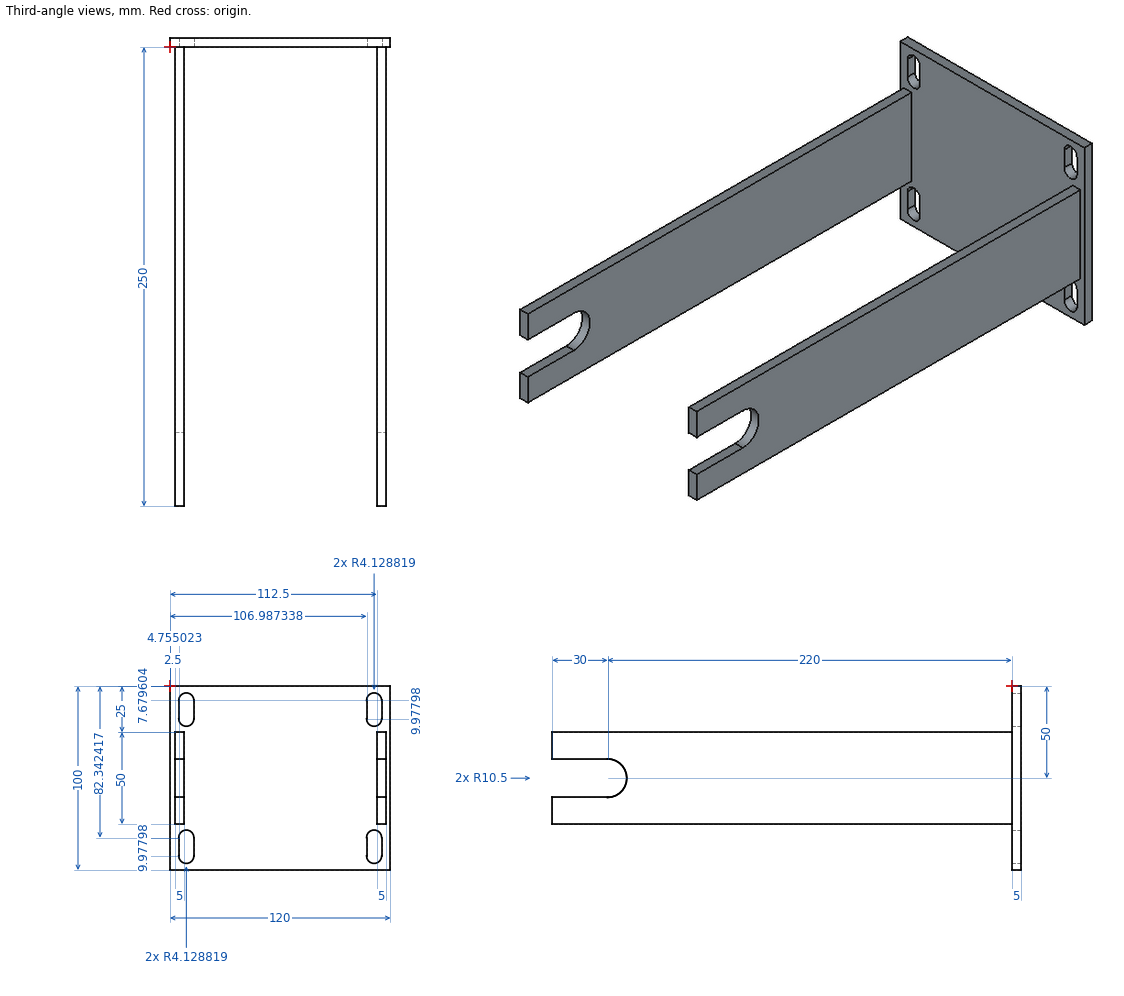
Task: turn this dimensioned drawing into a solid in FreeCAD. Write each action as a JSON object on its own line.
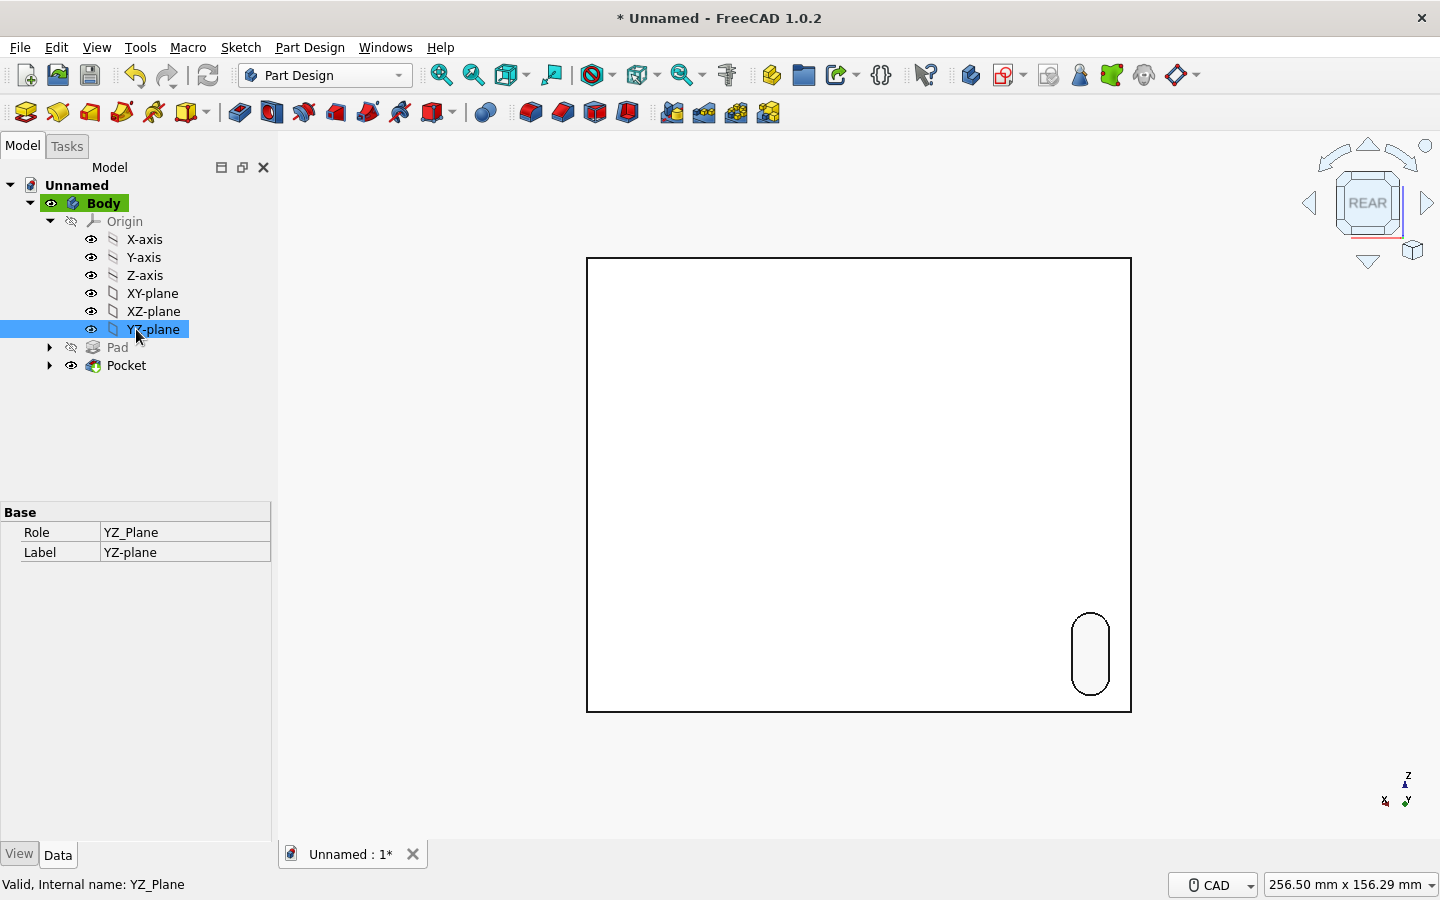
{"action": "left_click", "coordinate": [1176, 76]}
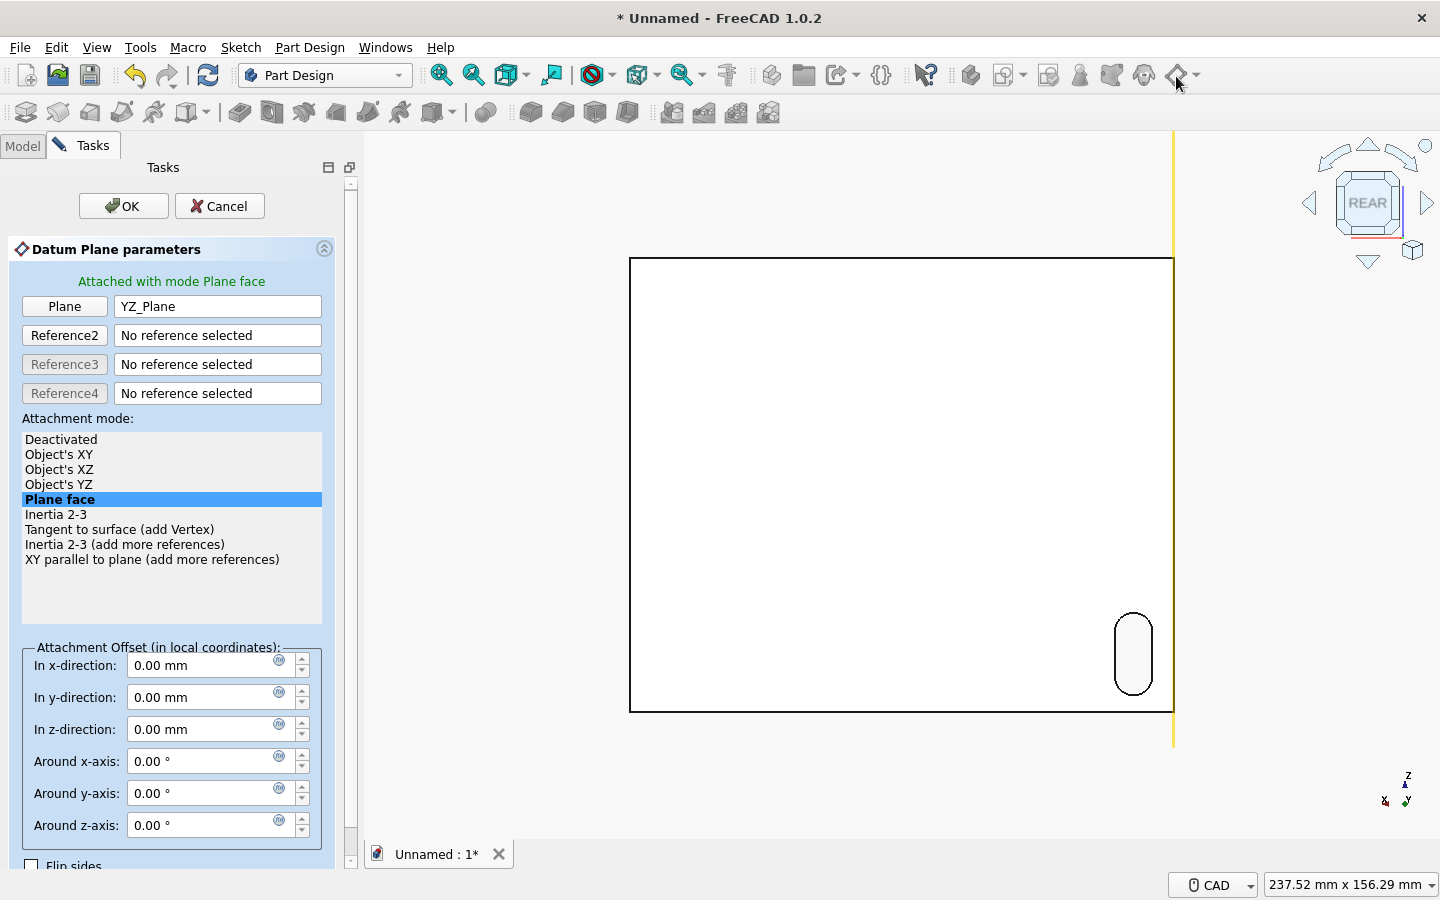
{"action": "triple_click", "coordinate": [210, 729]}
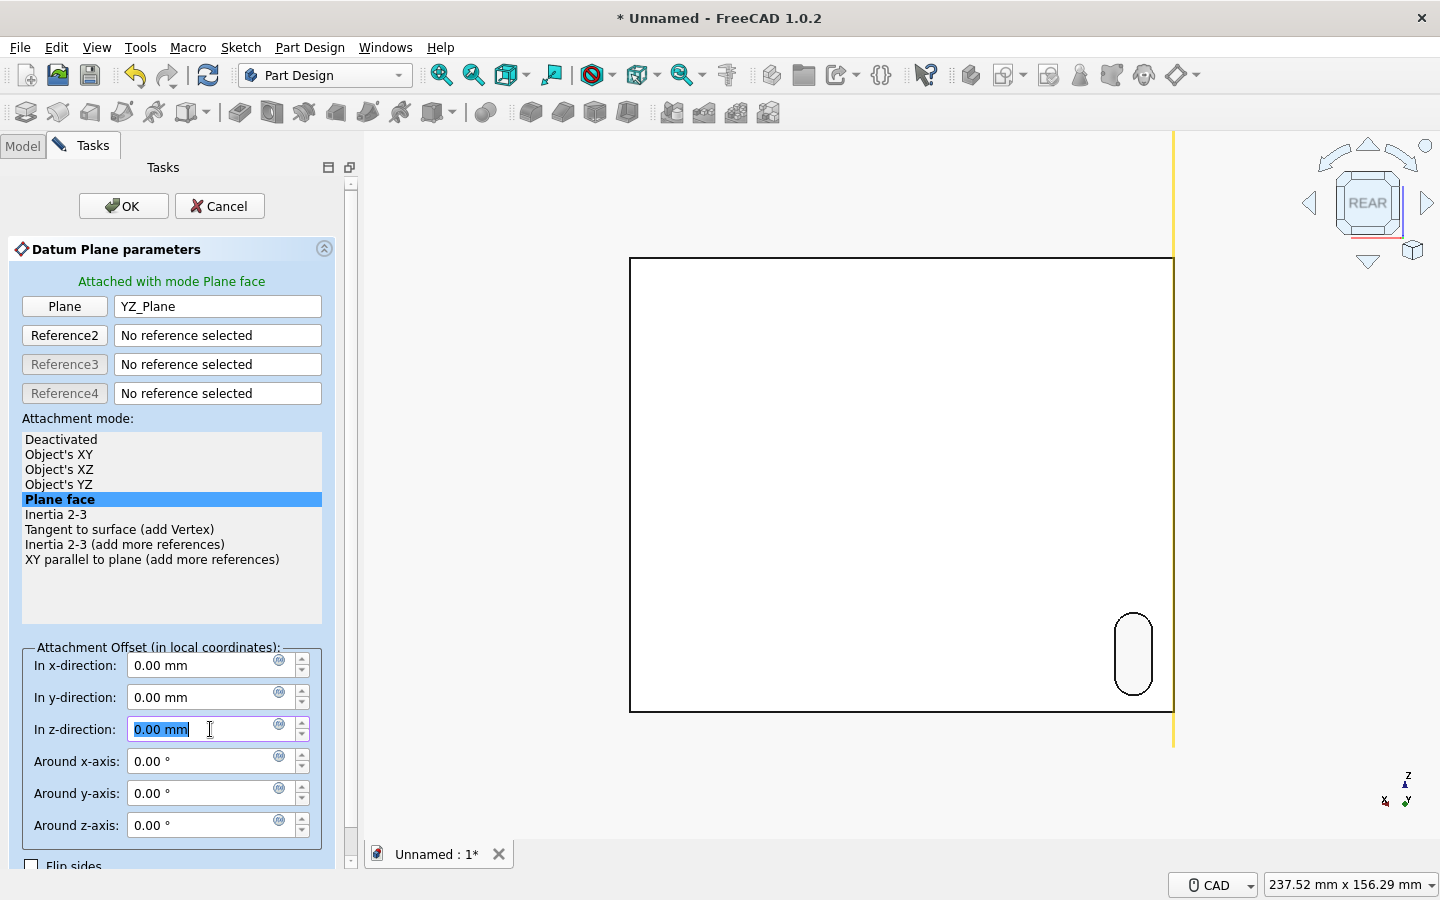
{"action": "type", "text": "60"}
{"action": "key", "text": "Tab"}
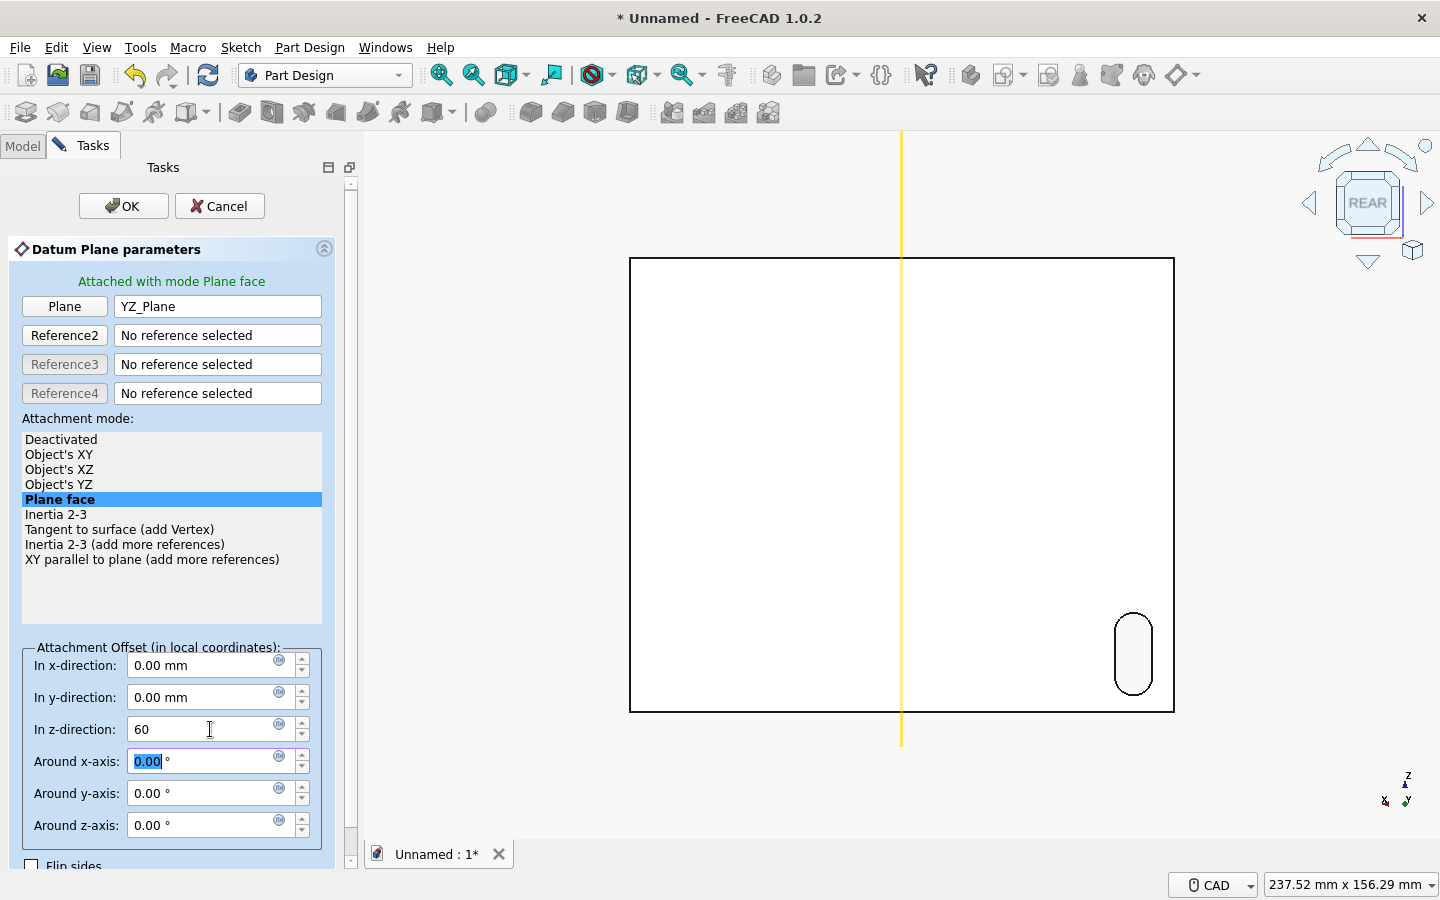
{"action": "left_click", "coordinate": [124, 206]}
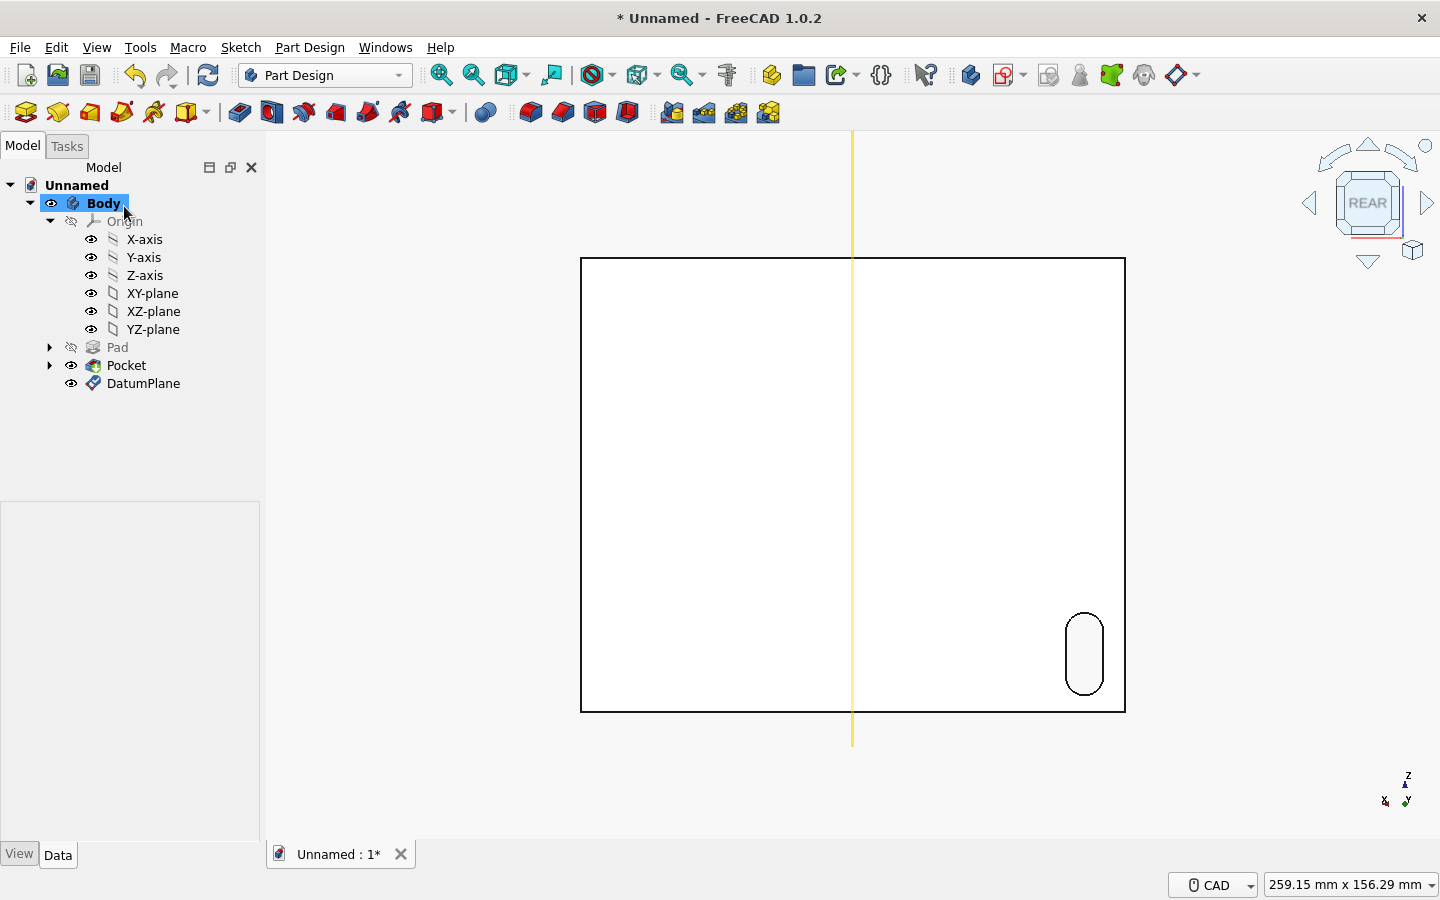
{"action": "left_click", "coordinate": [116, 365]}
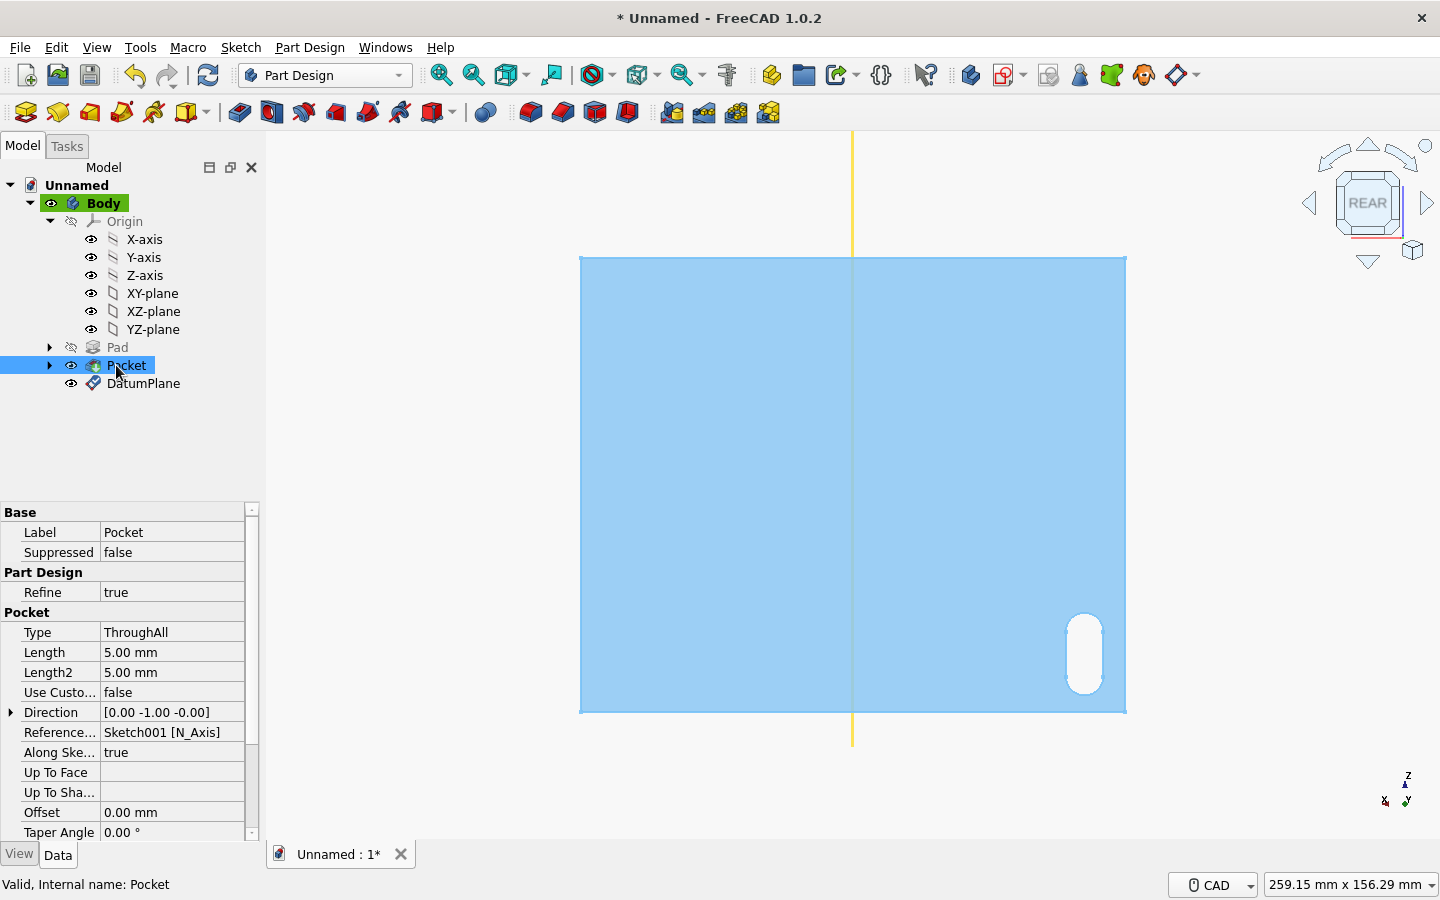
{"action": "left_click", "coordinate": [672, 112]}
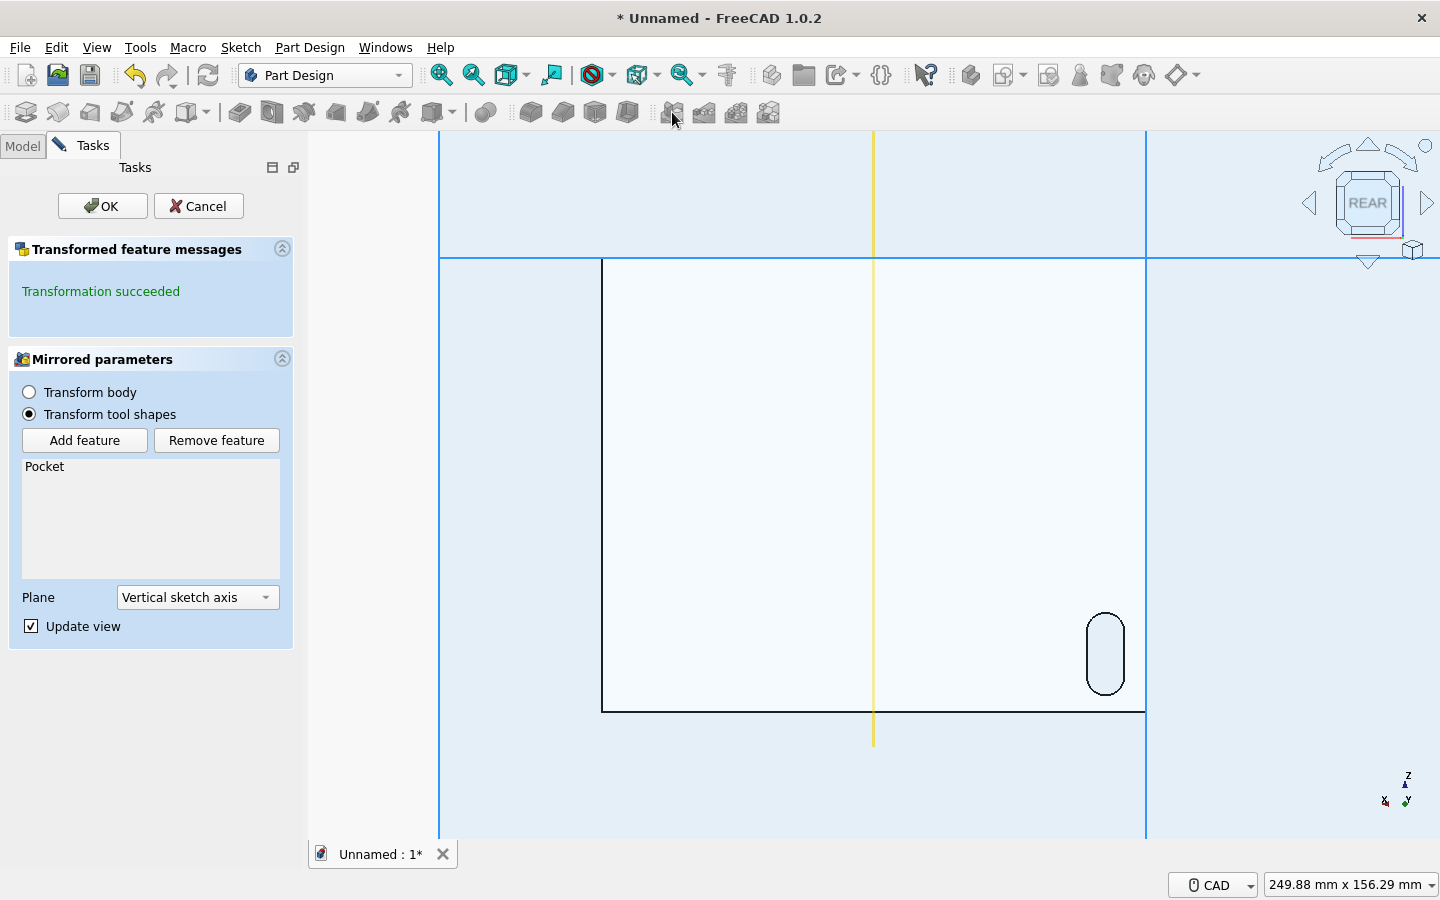
{"action": "left_click", "coordinate": [198, 598]}